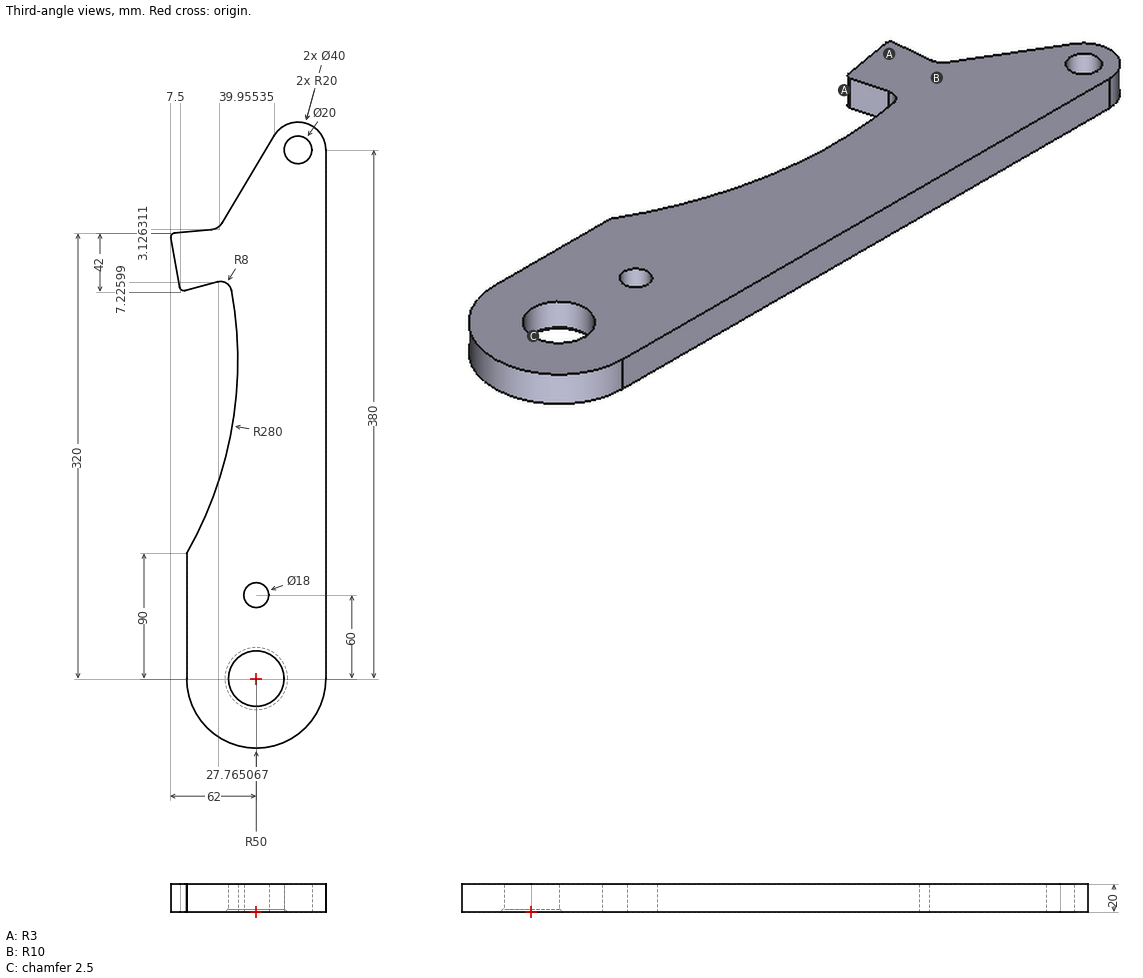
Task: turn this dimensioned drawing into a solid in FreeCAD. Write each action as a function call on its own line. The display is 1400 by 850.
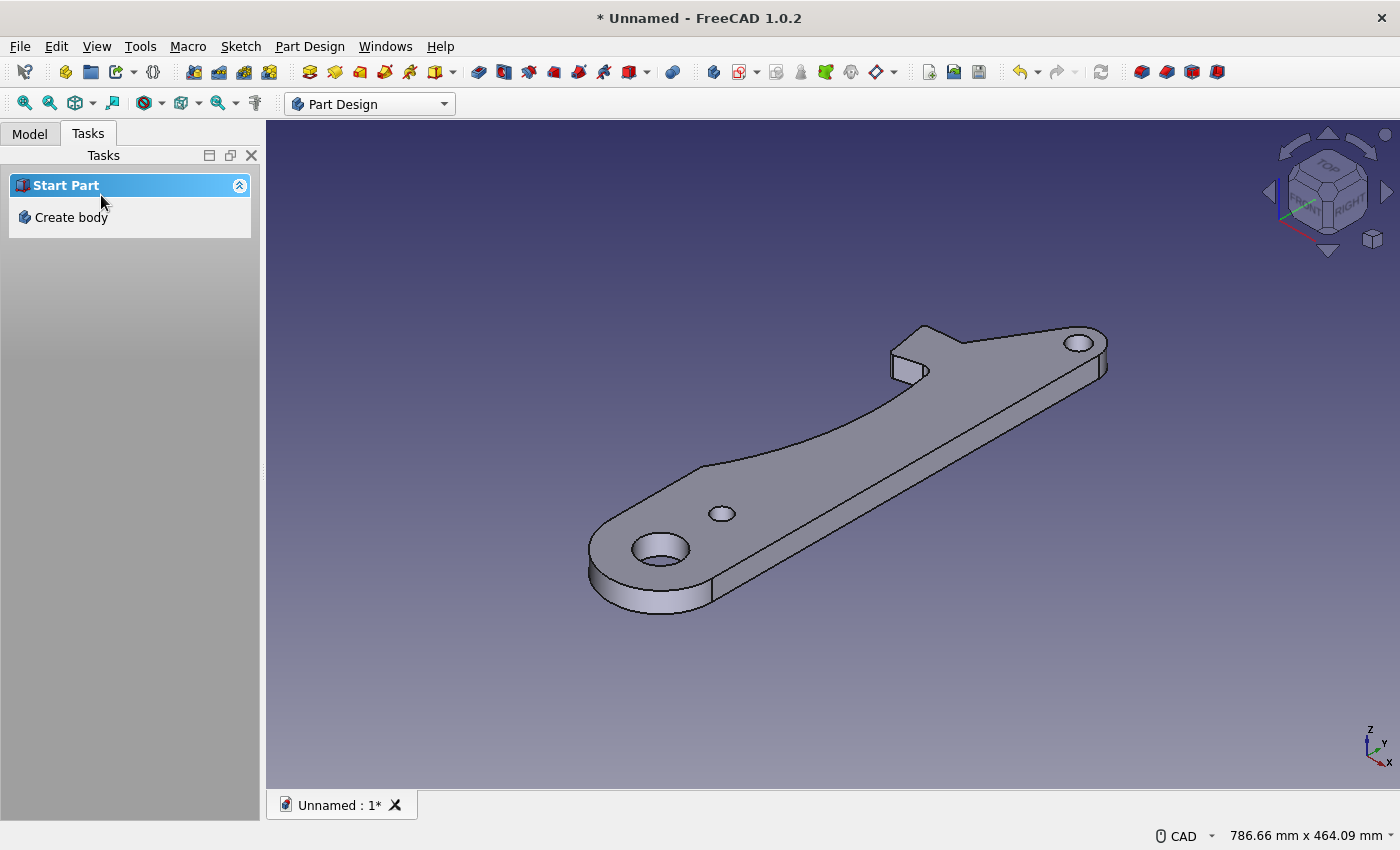
key(2)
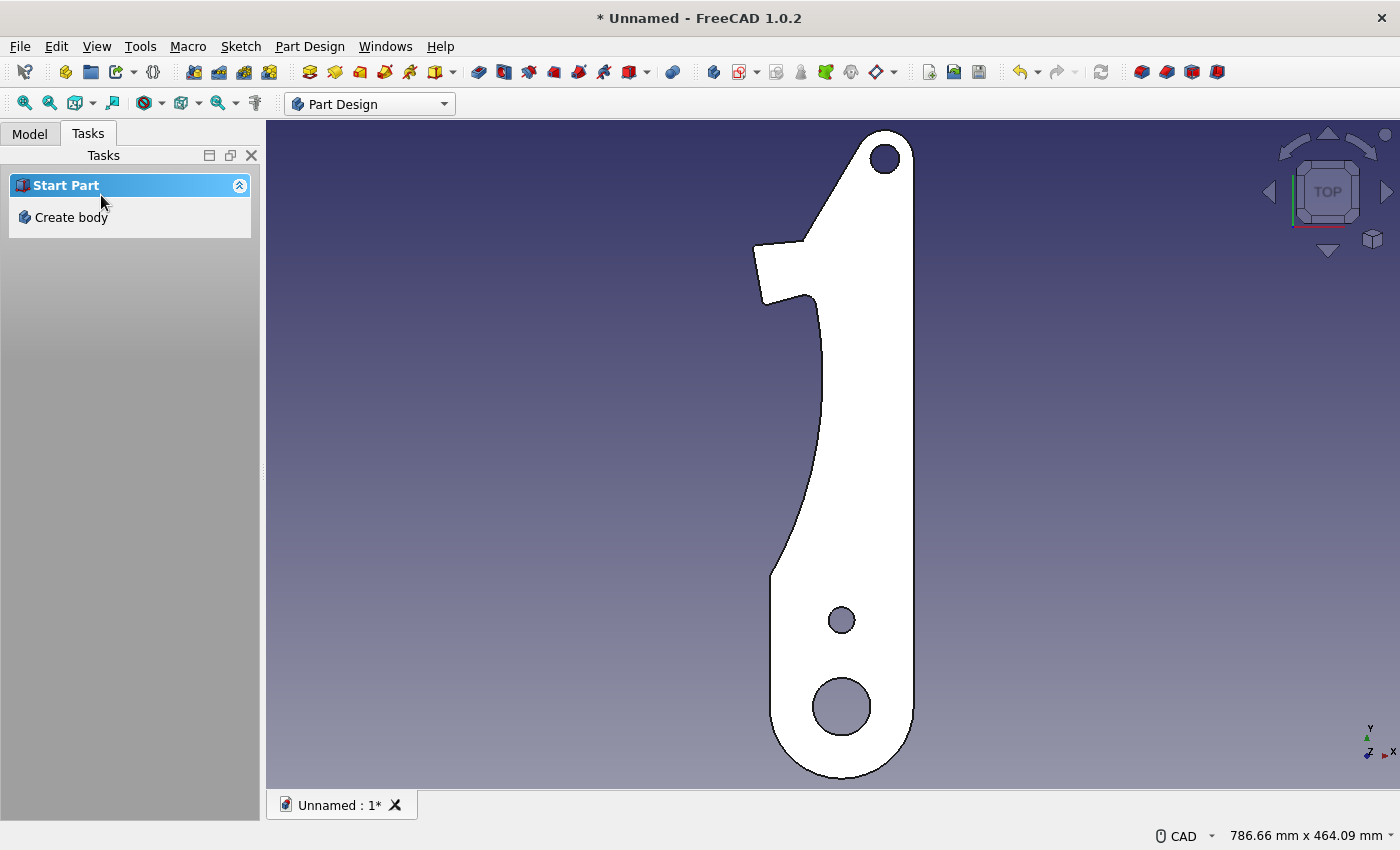
key(1)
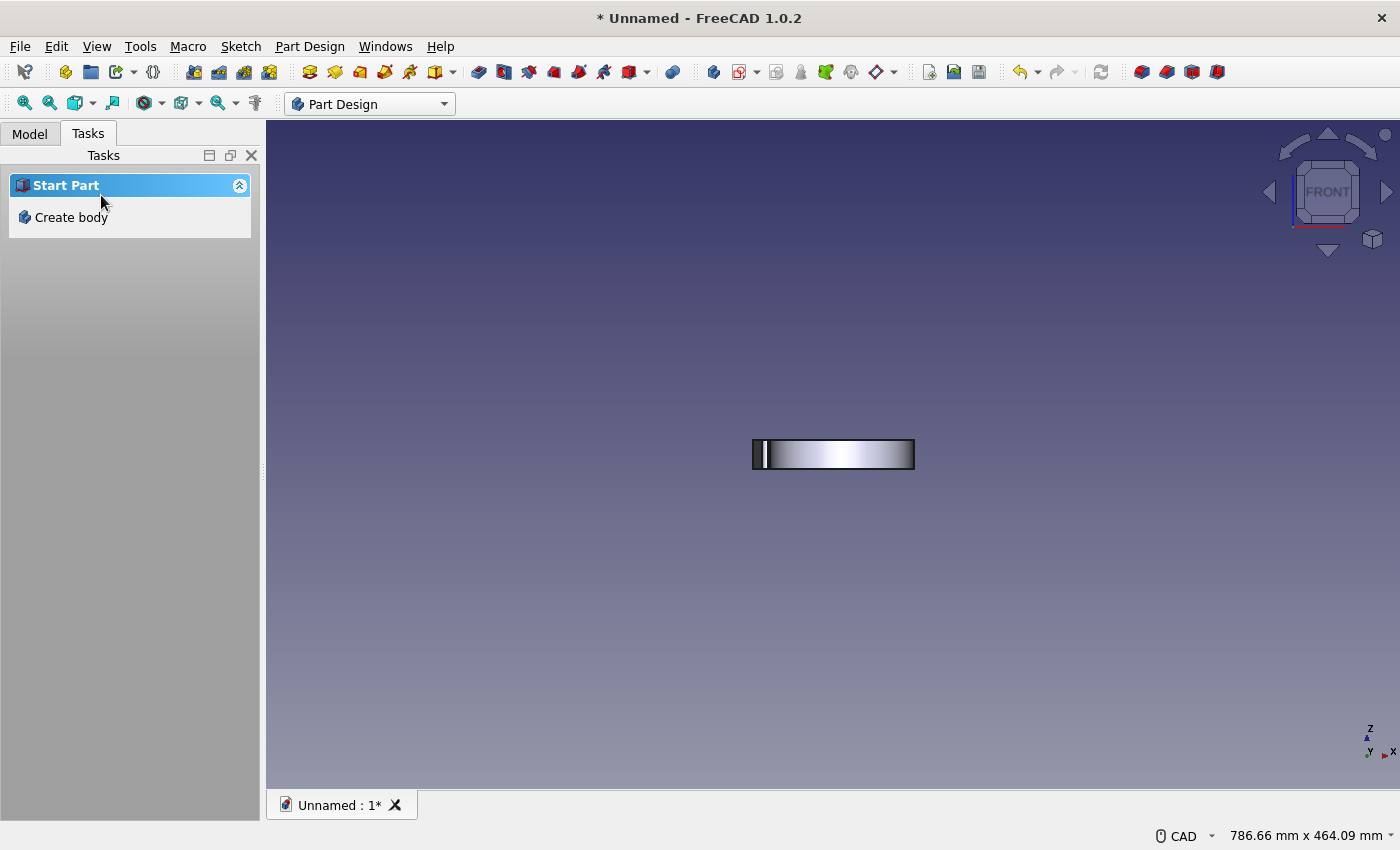
key(v)
key(f)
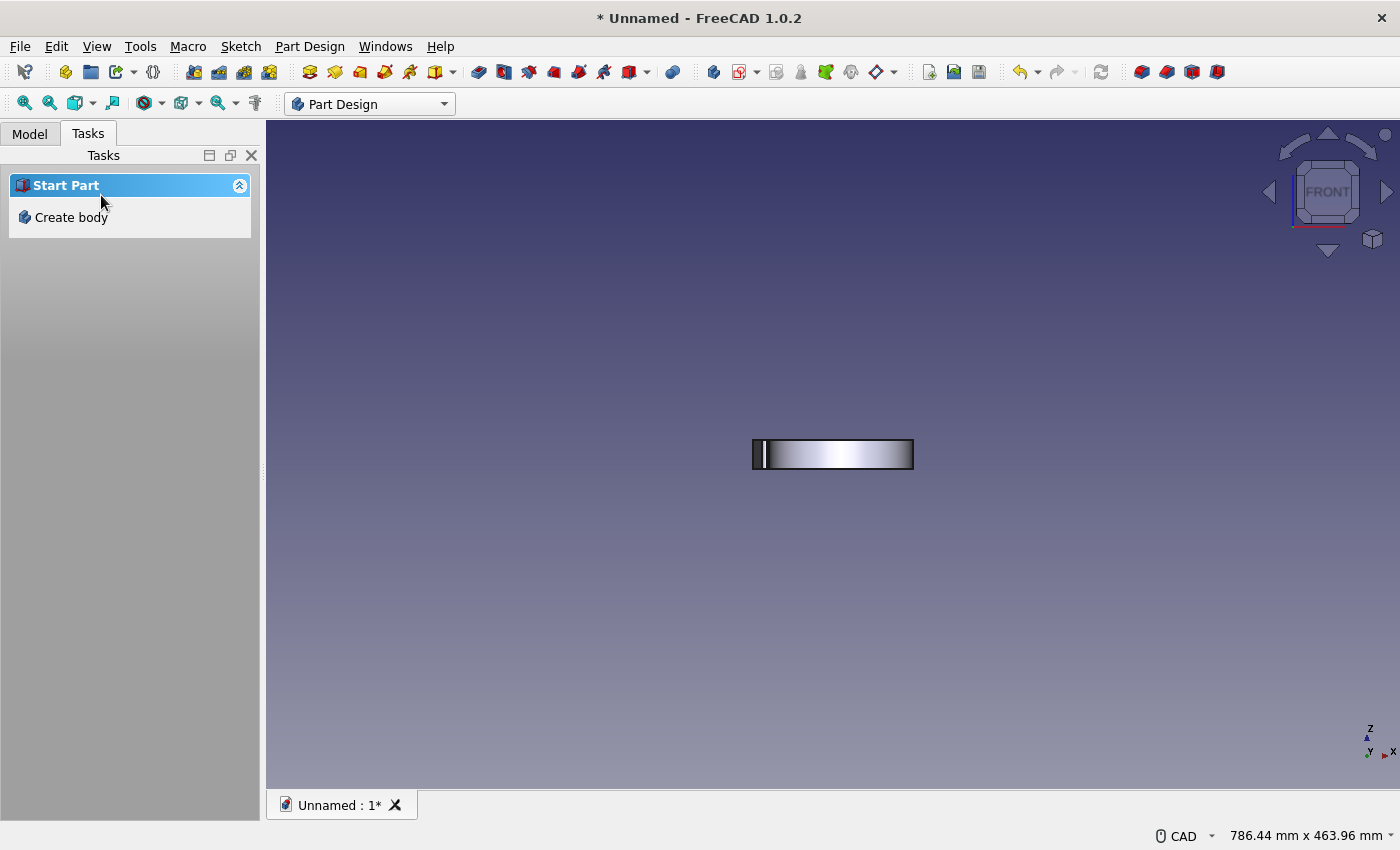
key(3)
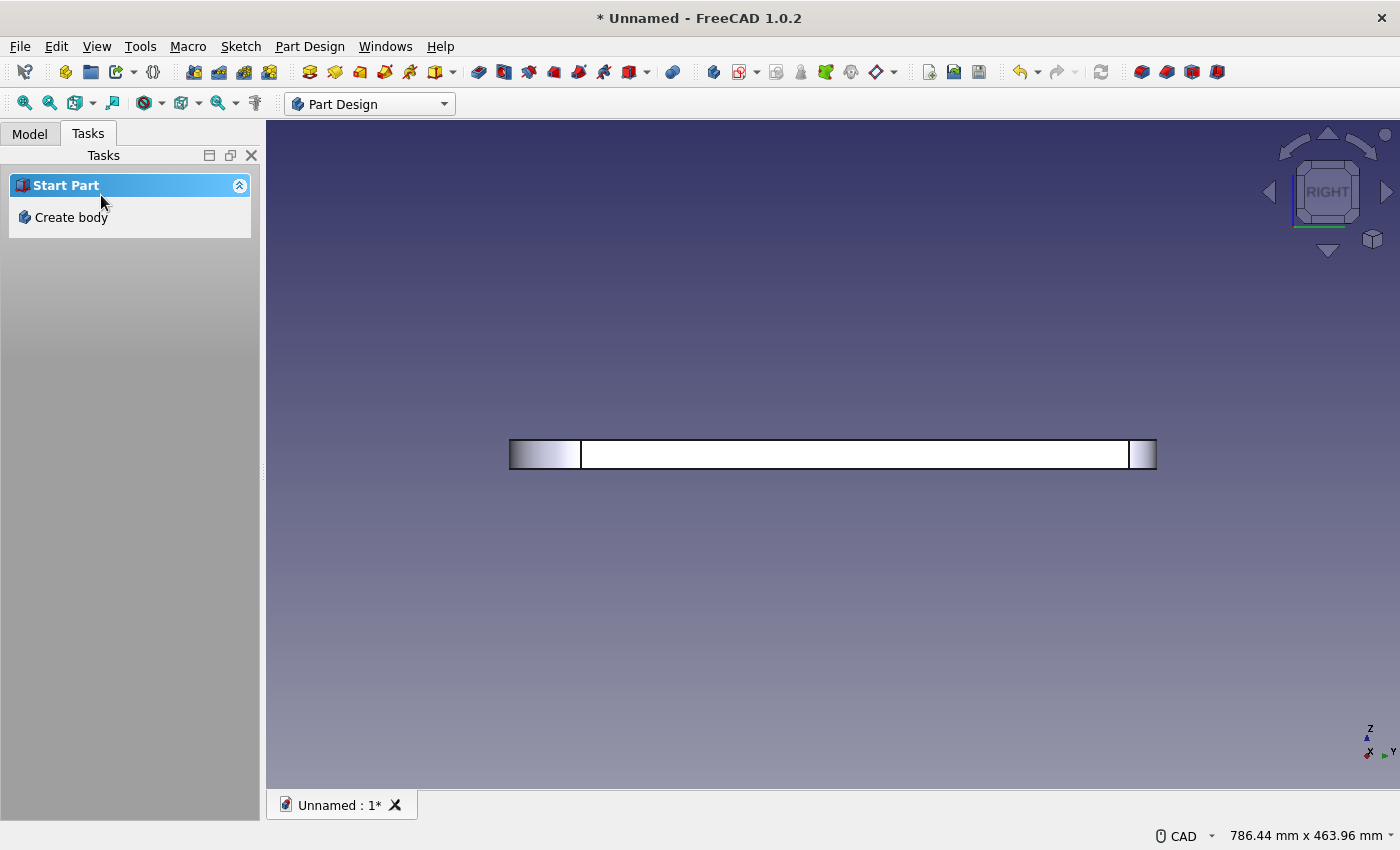
key(5)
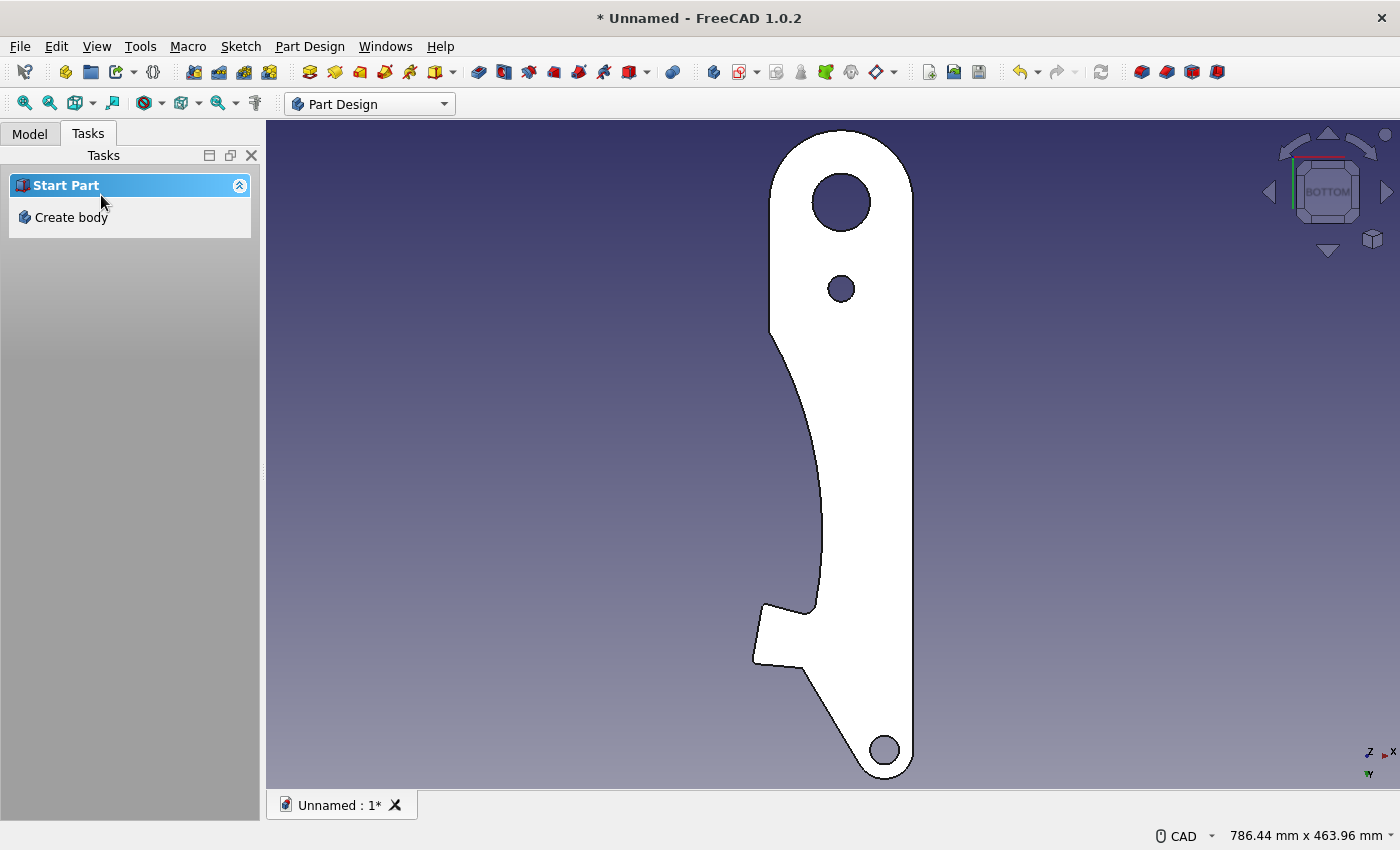
key(4)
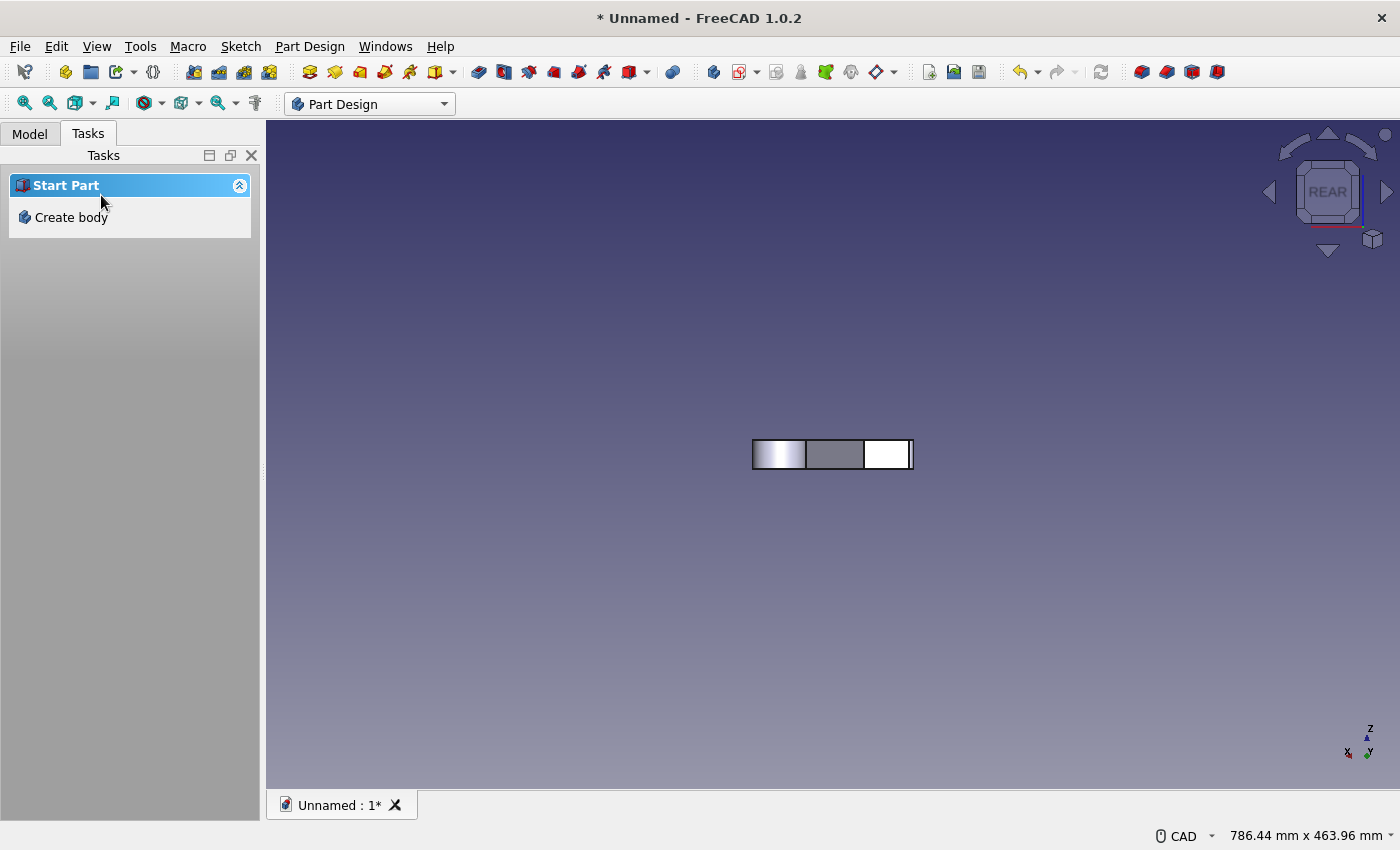
key(v)
key(f)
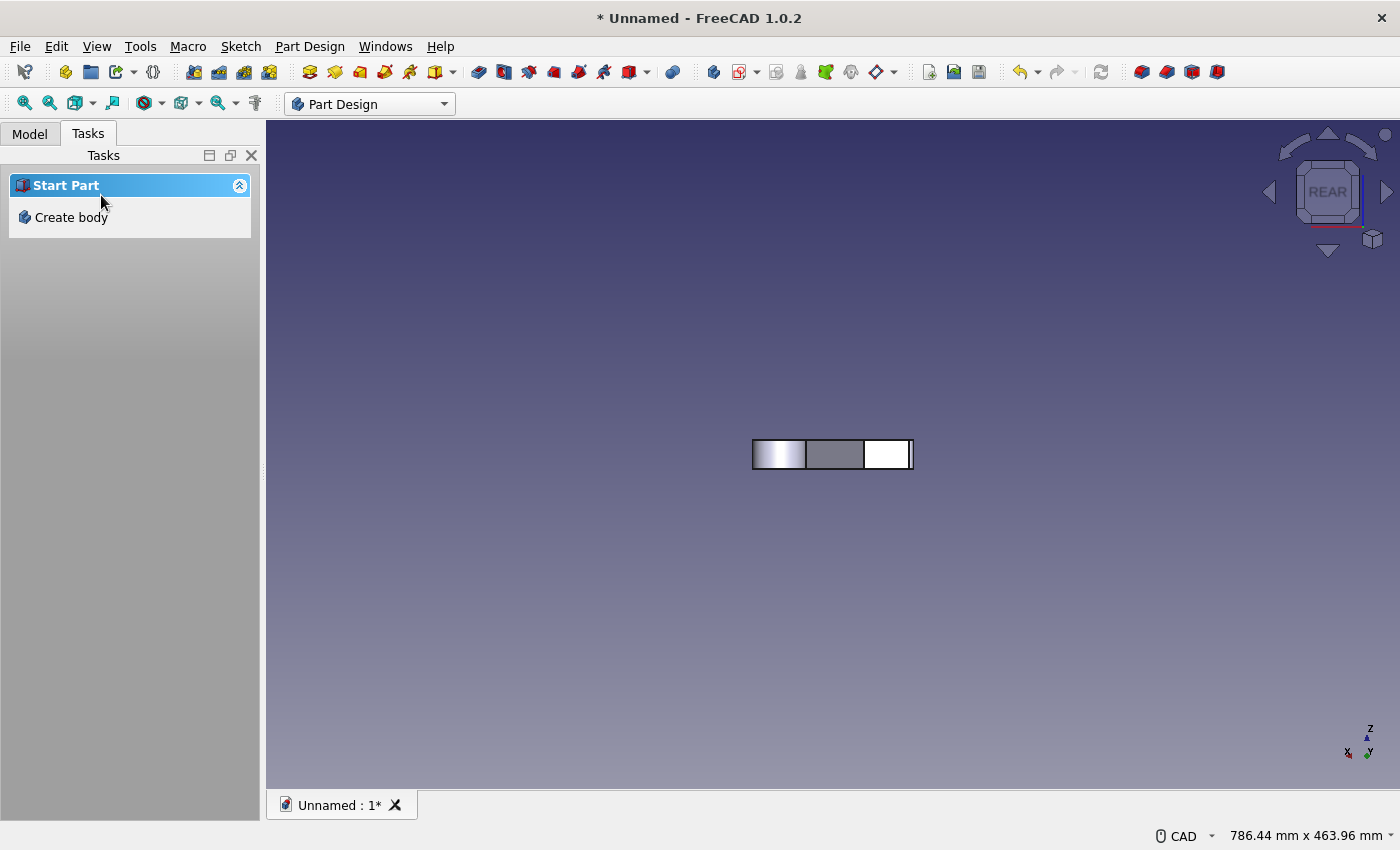
key(6)